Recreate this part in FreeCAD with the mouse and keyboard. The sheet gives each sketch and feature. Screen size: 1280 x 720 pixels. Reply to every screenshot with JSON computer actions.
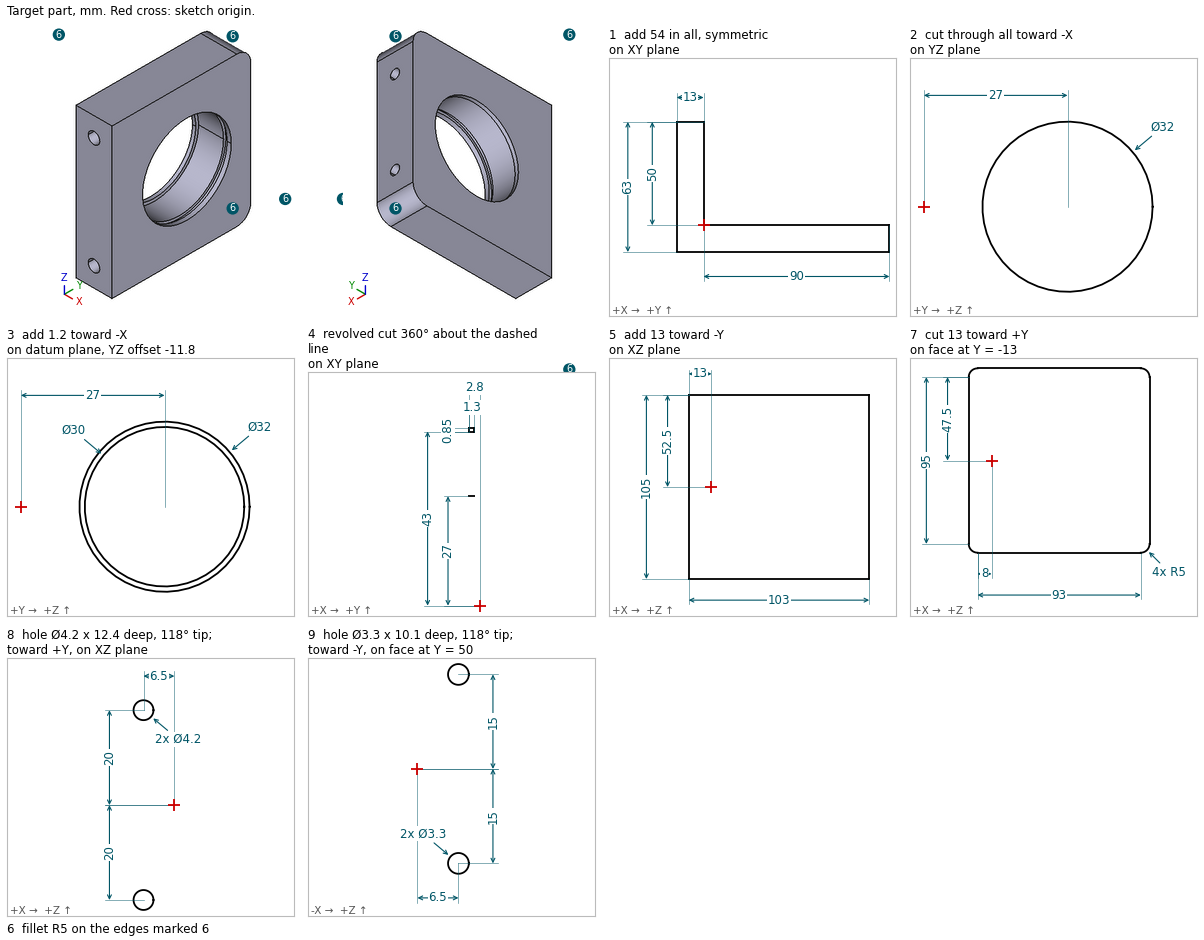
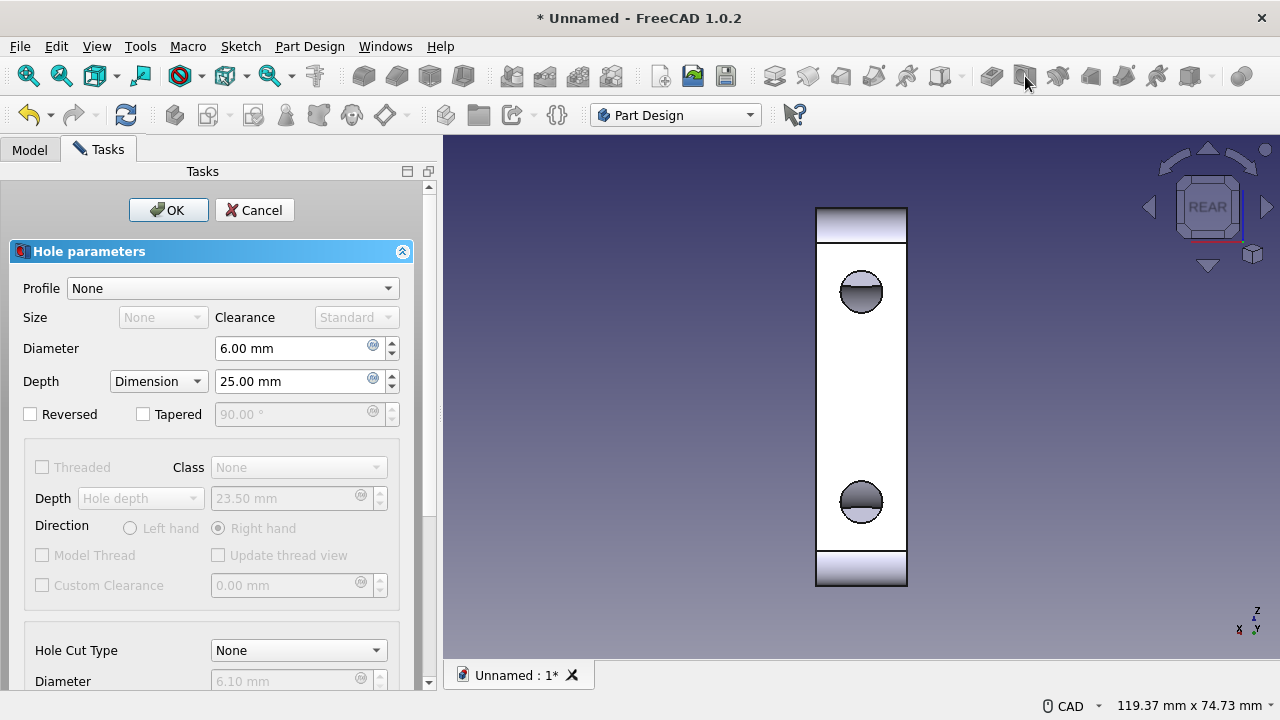
{"action": "triple_click", "coordinate": [300, 348]}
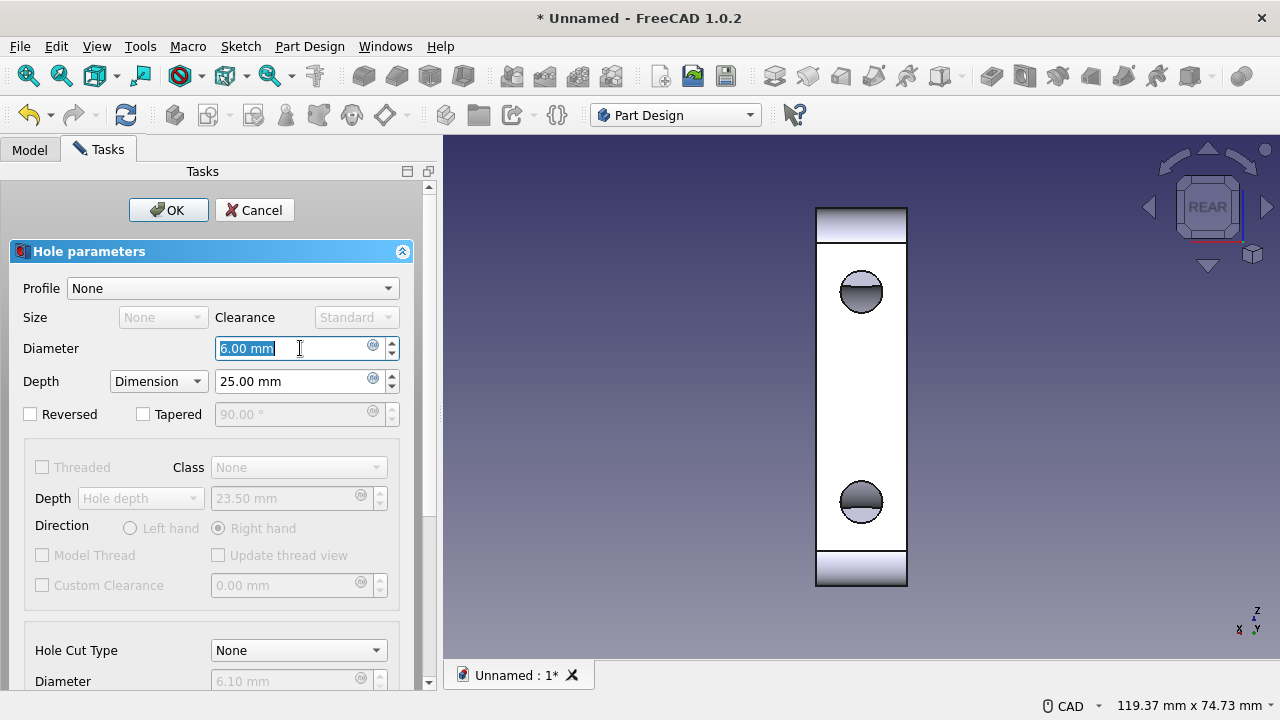
{"action": "type", "text": "3.3"}
{"action": "key", "text": "Tab"}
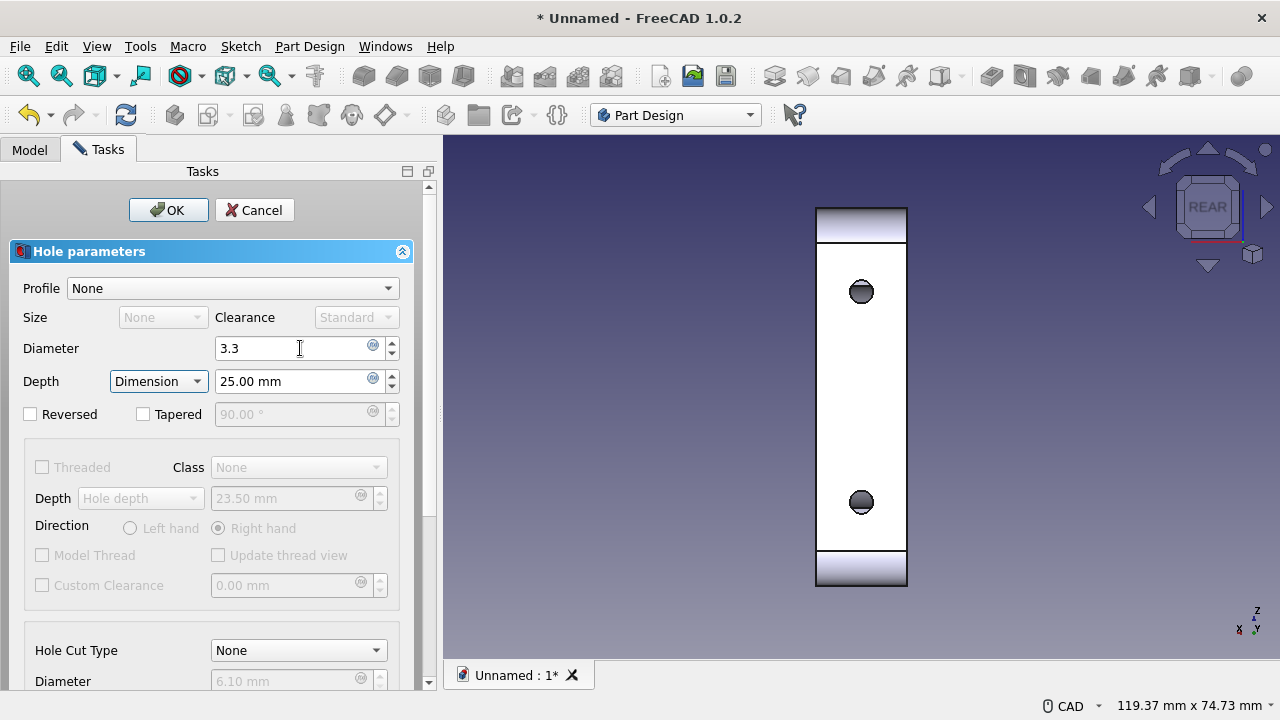
{"action": "triple_click", "coordinate": [300, 382]}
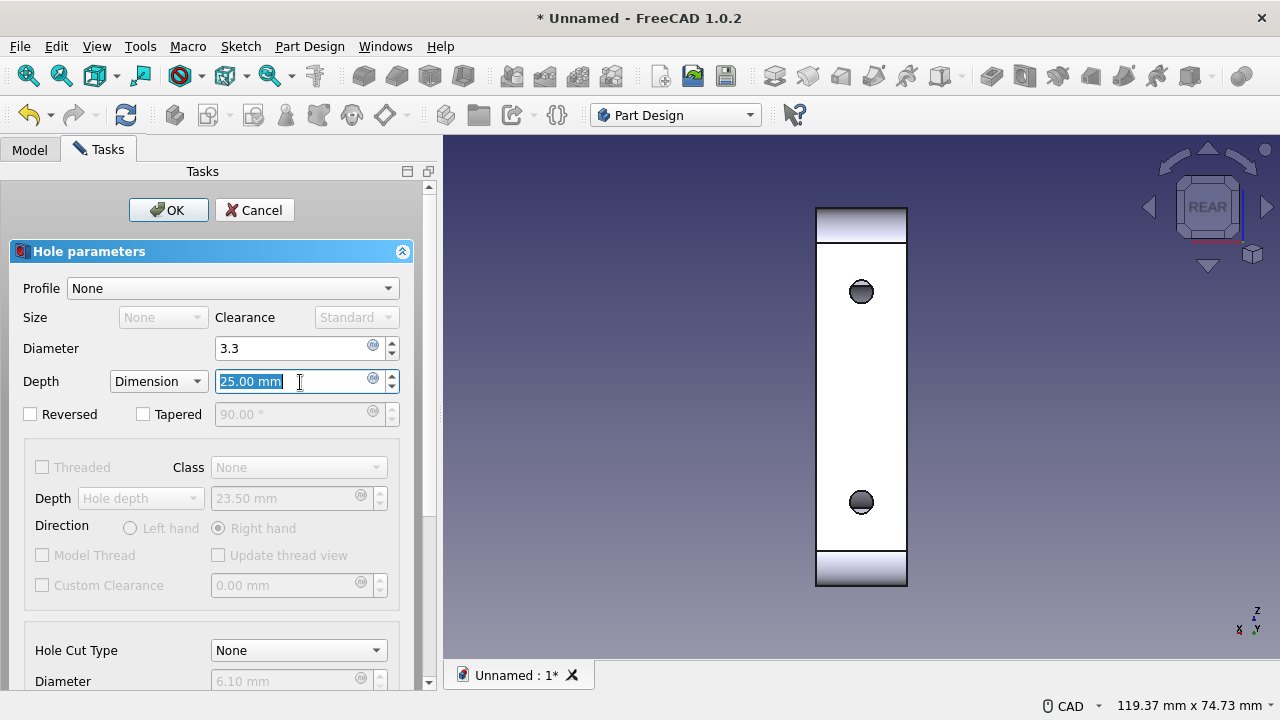
{"action": "type", "text": "10.1"}
{"action": "key", "text": "Tab"}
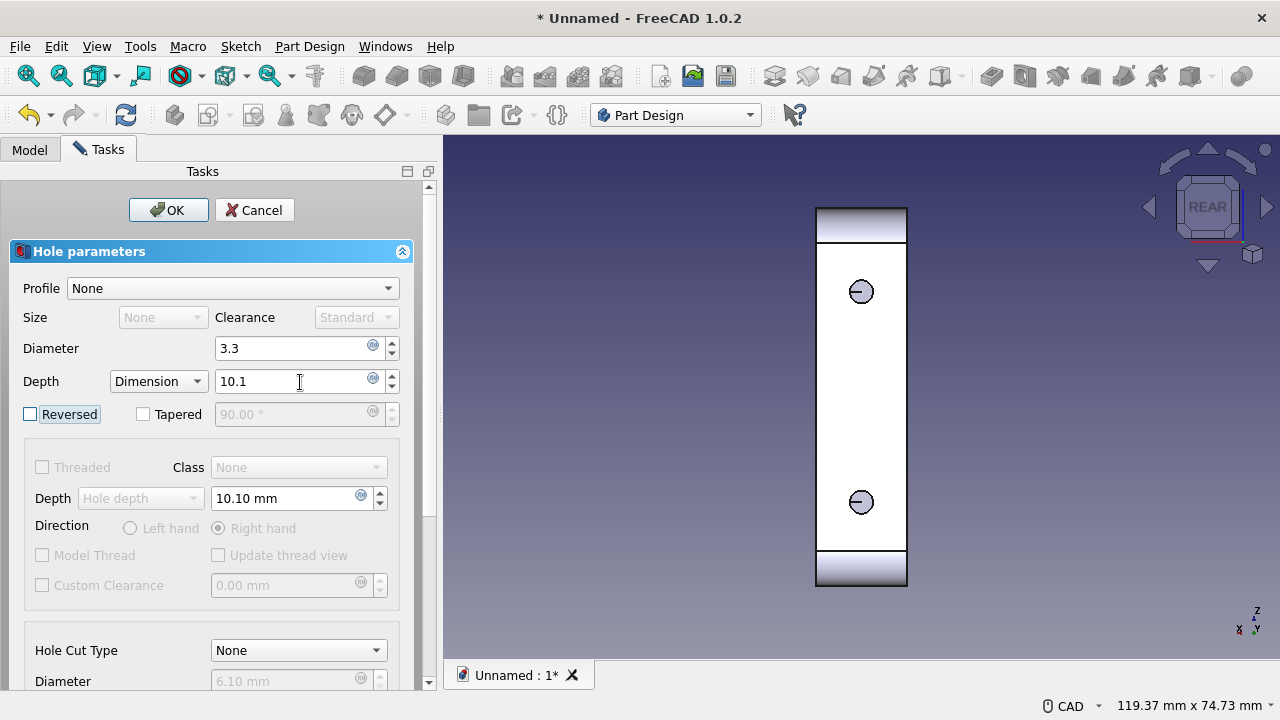
{"action": "left_click", "coordinate": [169, 210]}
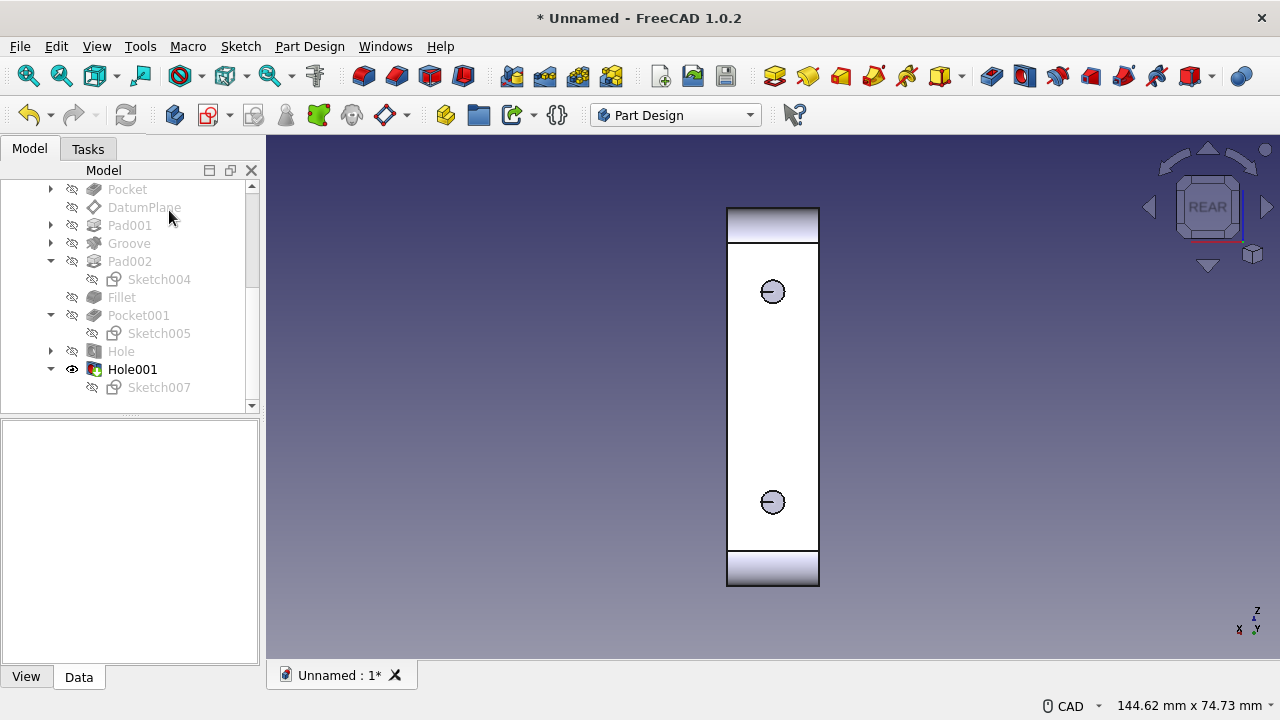
{"action": "key", "text": "0"}